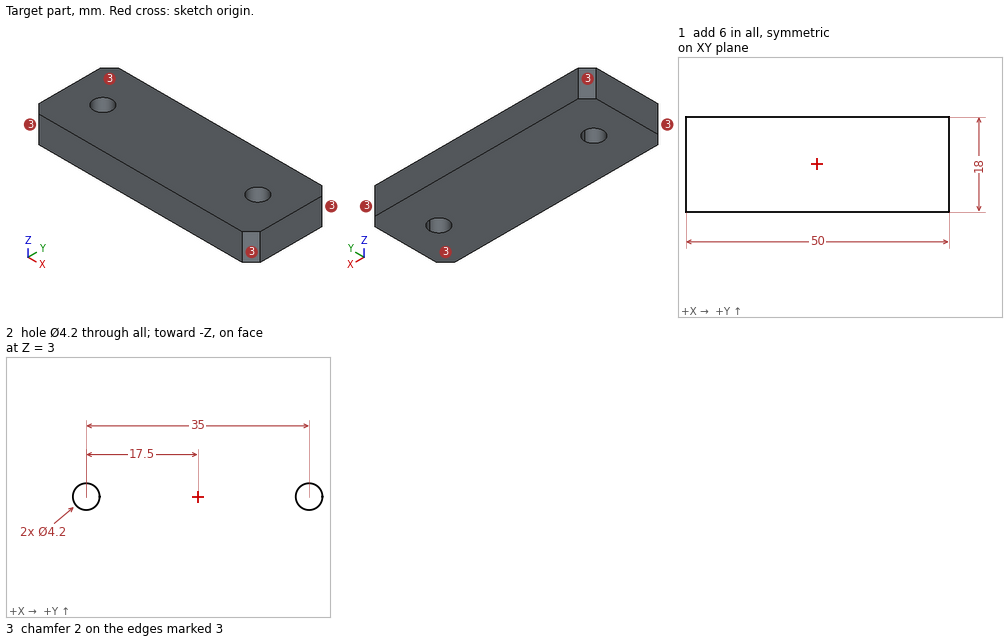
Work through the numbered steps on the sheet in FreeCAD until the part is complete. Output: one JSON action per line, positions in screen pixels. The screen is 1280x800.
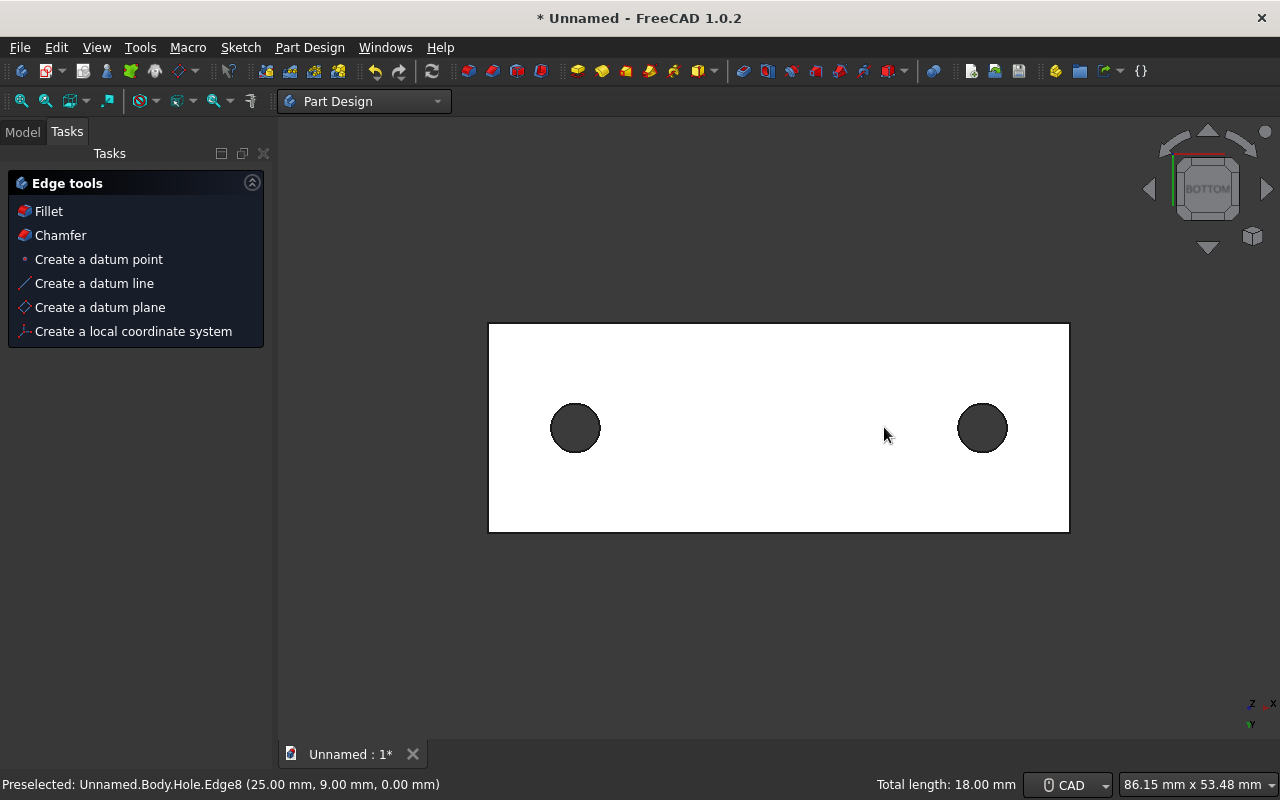
{"action": "key", "text": "4"}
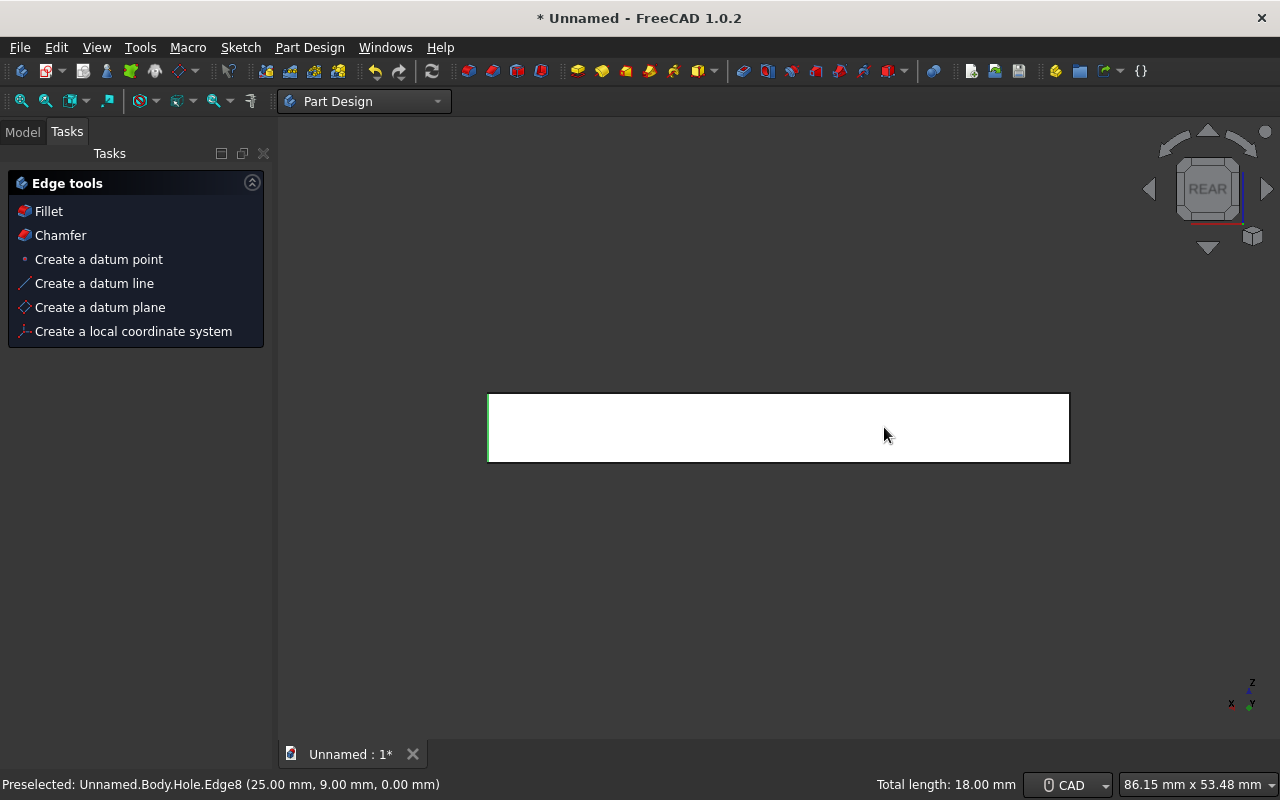
{"action": "left_click", "coordinate": [1070, 427], "text": "ctrl"}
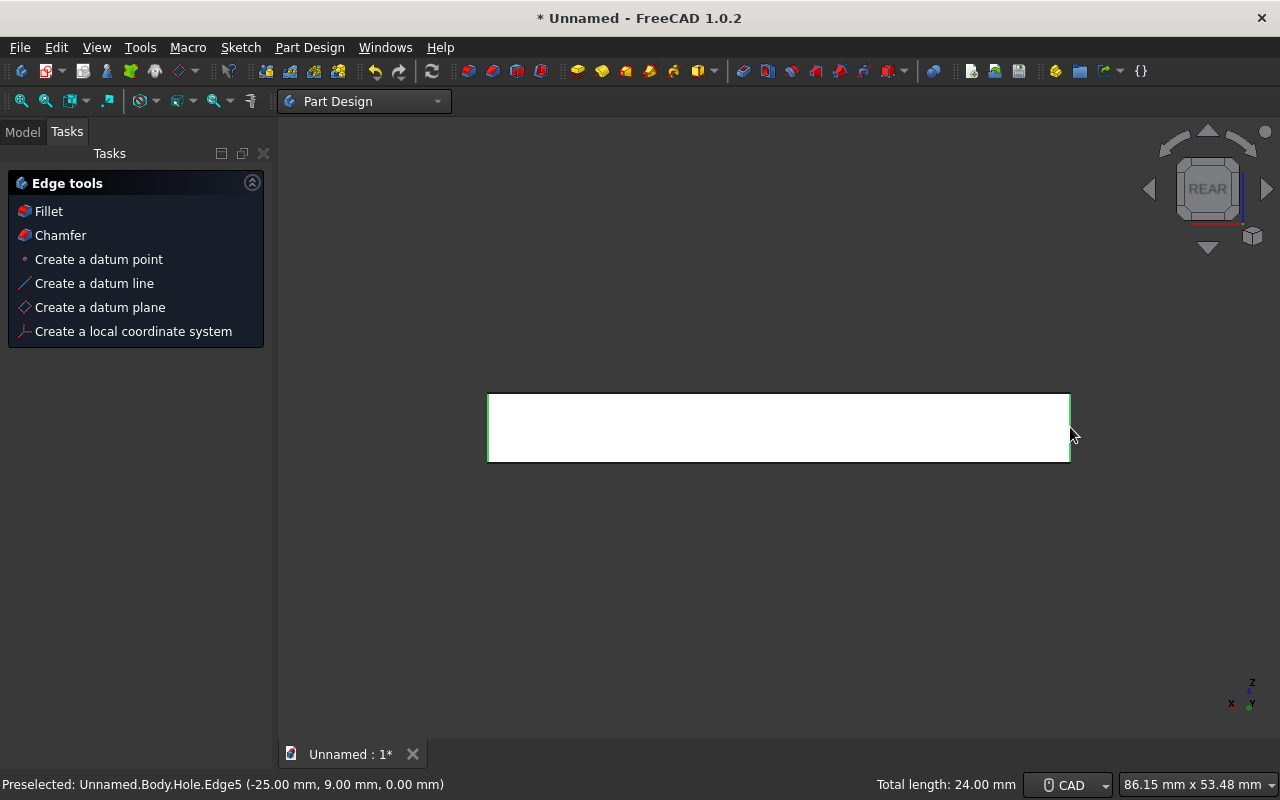
{"action": "left_click", "coordinate": [494, 72]}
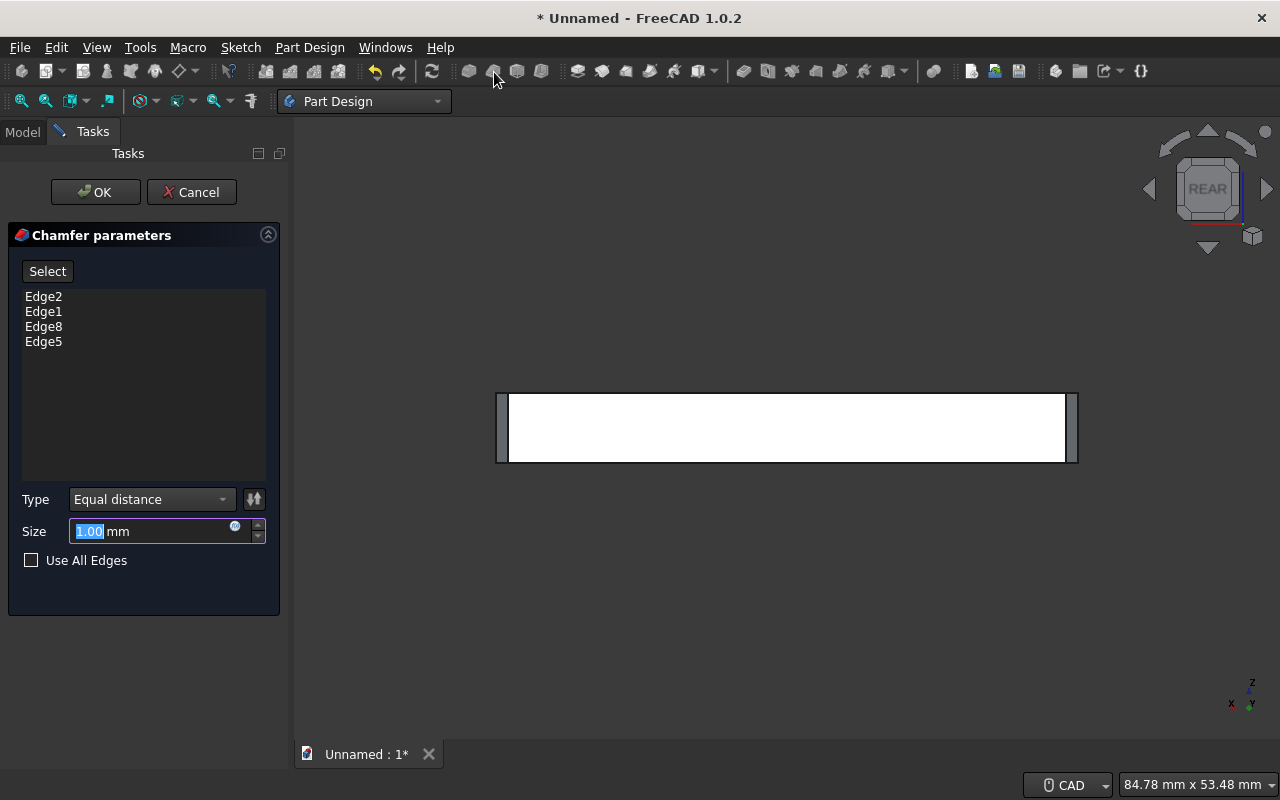
{"action": "type", "text": "2"}
{"action": "key", "text": "Tab"}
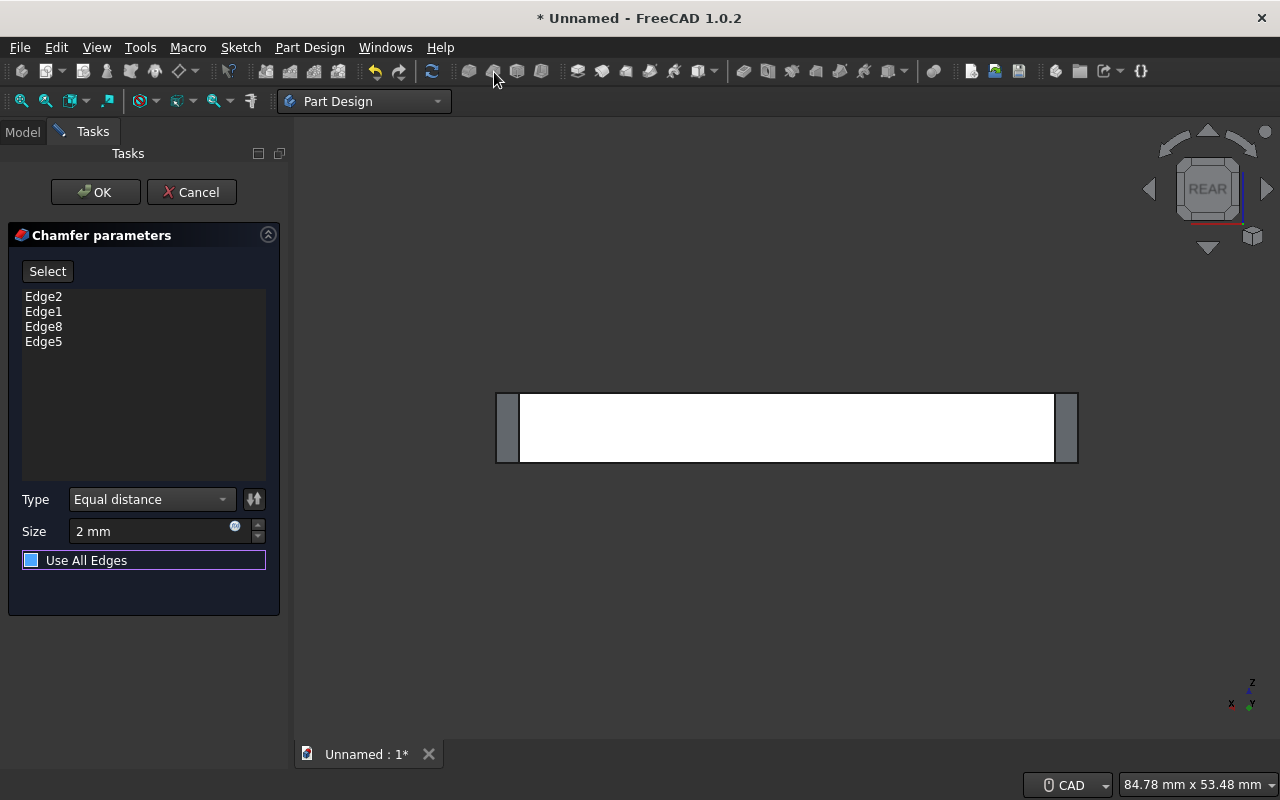
{"action": "left_click", "coordinate": [96, 192]}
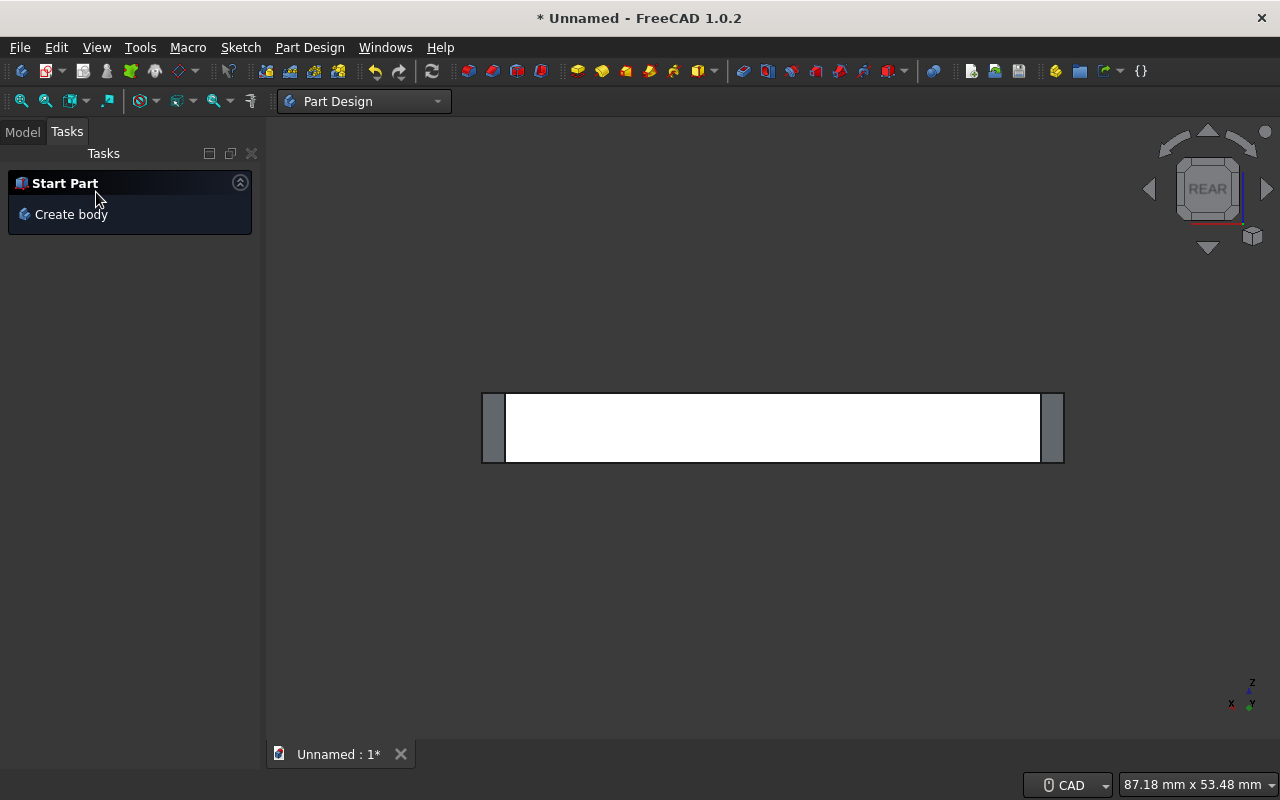
{"action": "key", "text": "0"}